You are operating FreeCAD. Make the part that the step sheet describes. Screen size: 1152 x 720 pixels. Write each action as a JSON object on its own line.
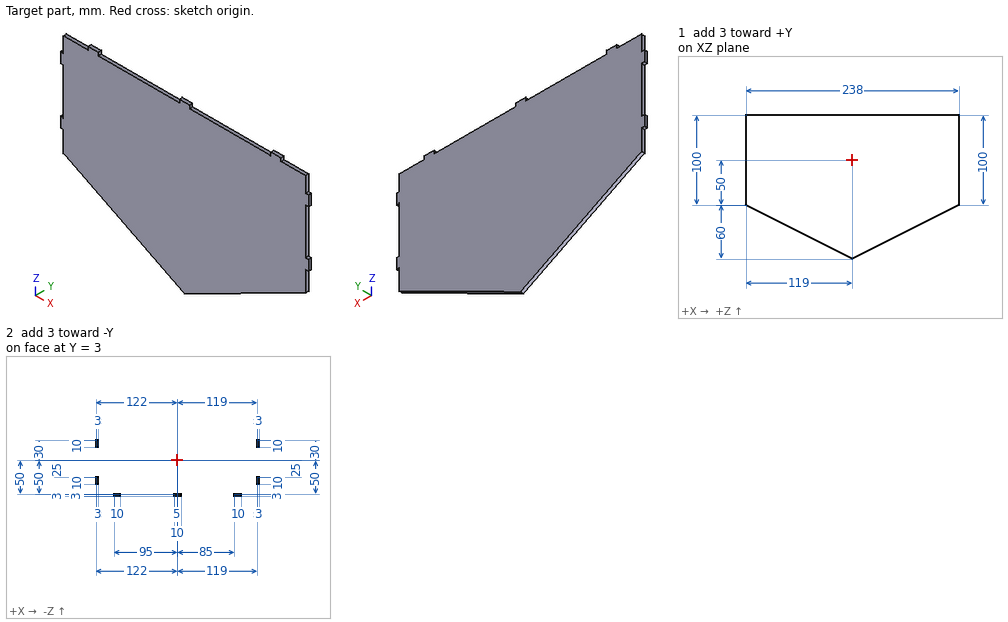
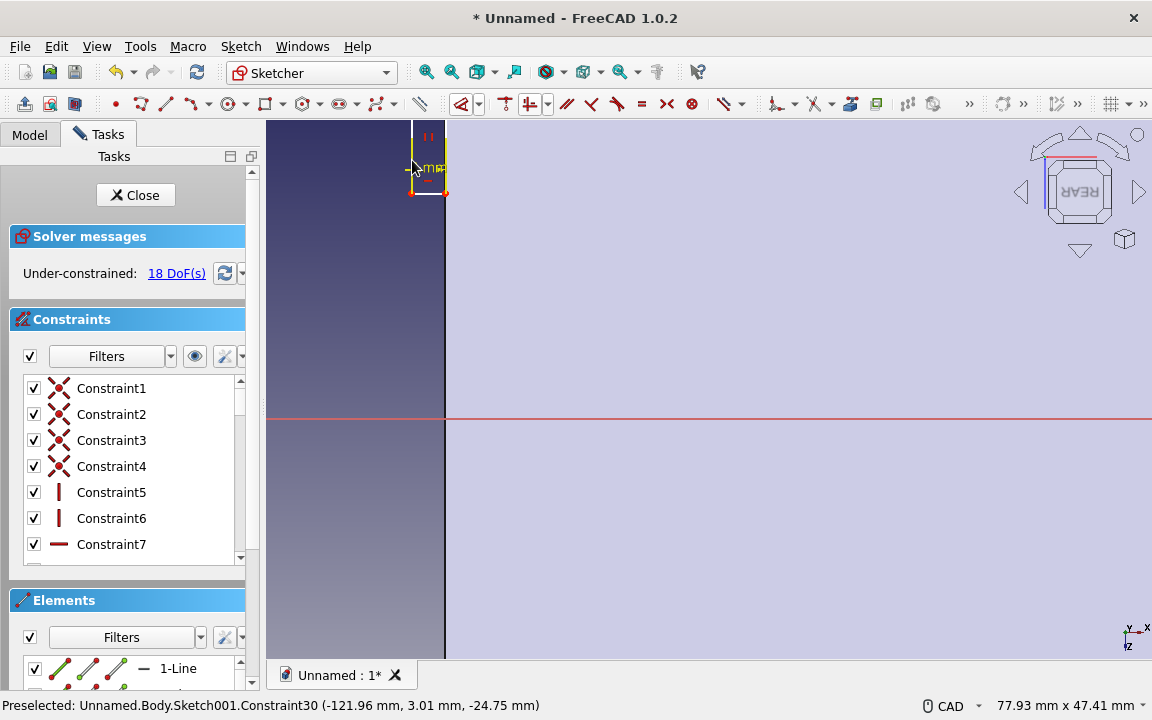
{"action": "left_click", "coordinate": [412, 159]}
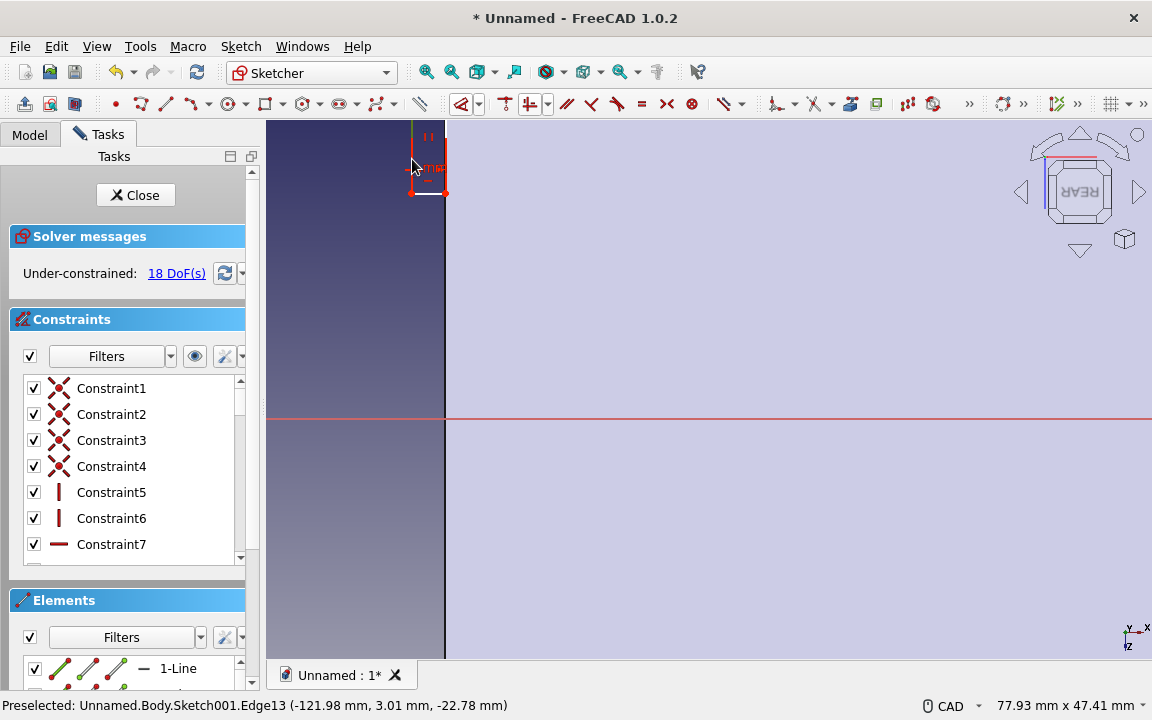
{"action": "key", "text": "i"}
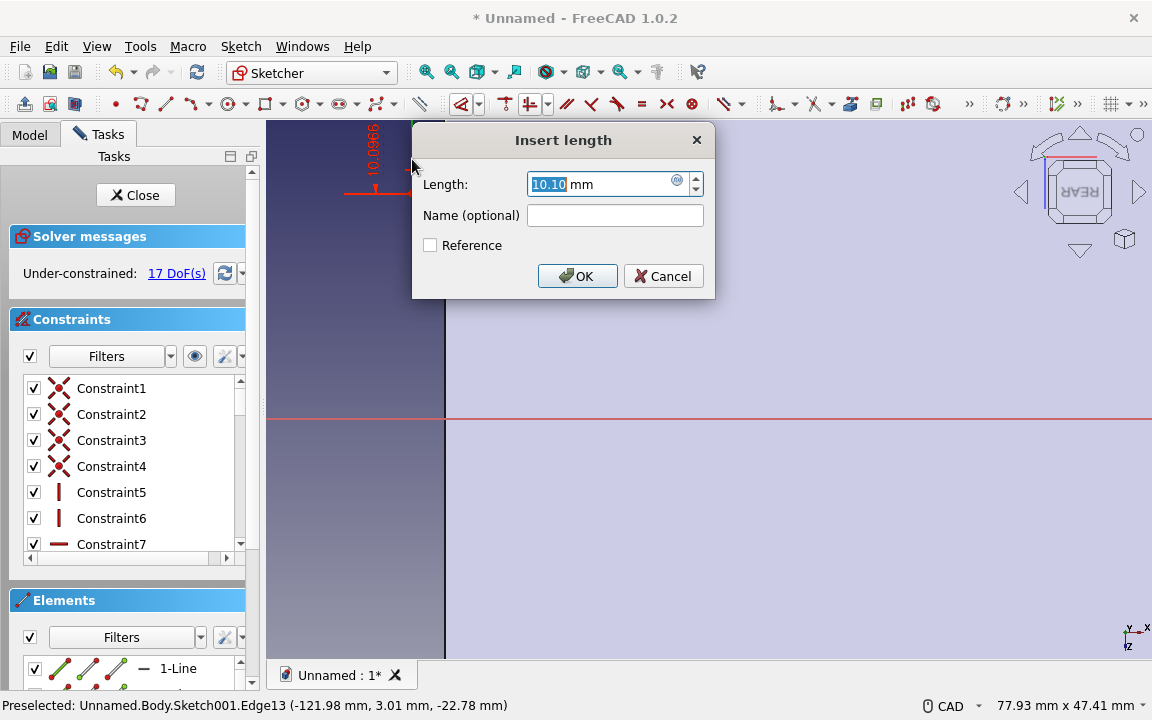
{"action": "type", "text": "10"}
{"action": "key", "text": "Return"}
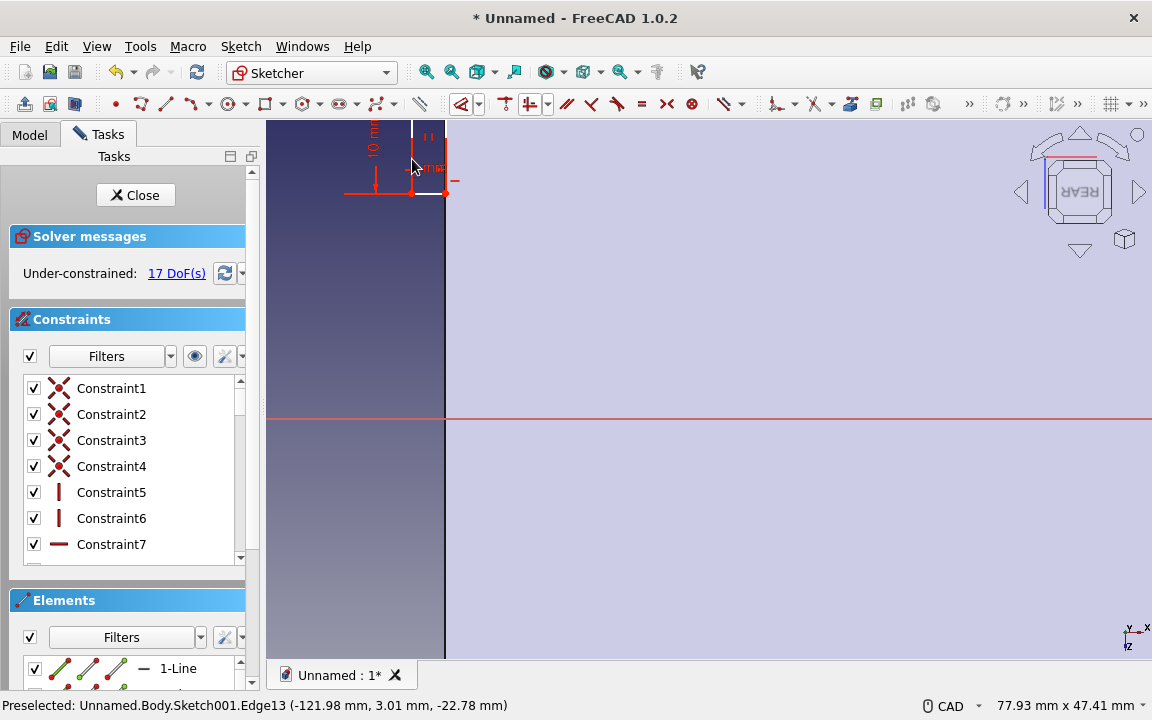
{"action": "scroll", "coordinate": [411, 358], "scroll_direction": "down", "scroll_amount": 9}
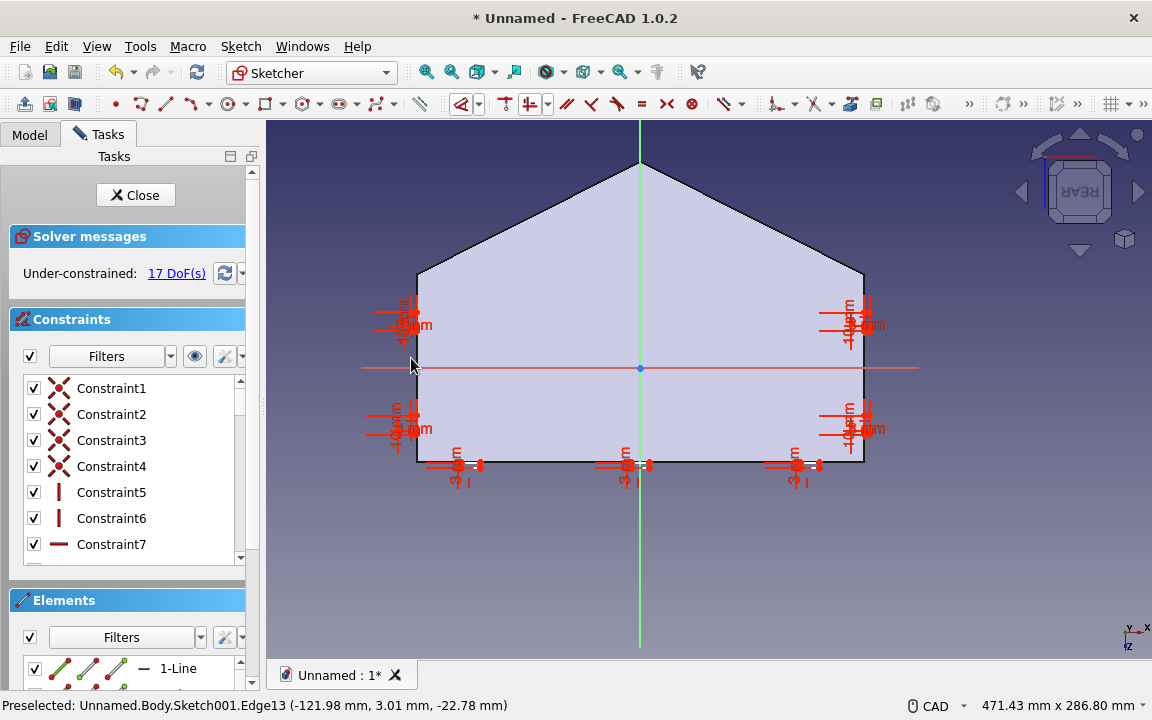
{"action": "scroll", "coordinate": [468, 468], "scroll_direction": "up", "scroll_amount": 5}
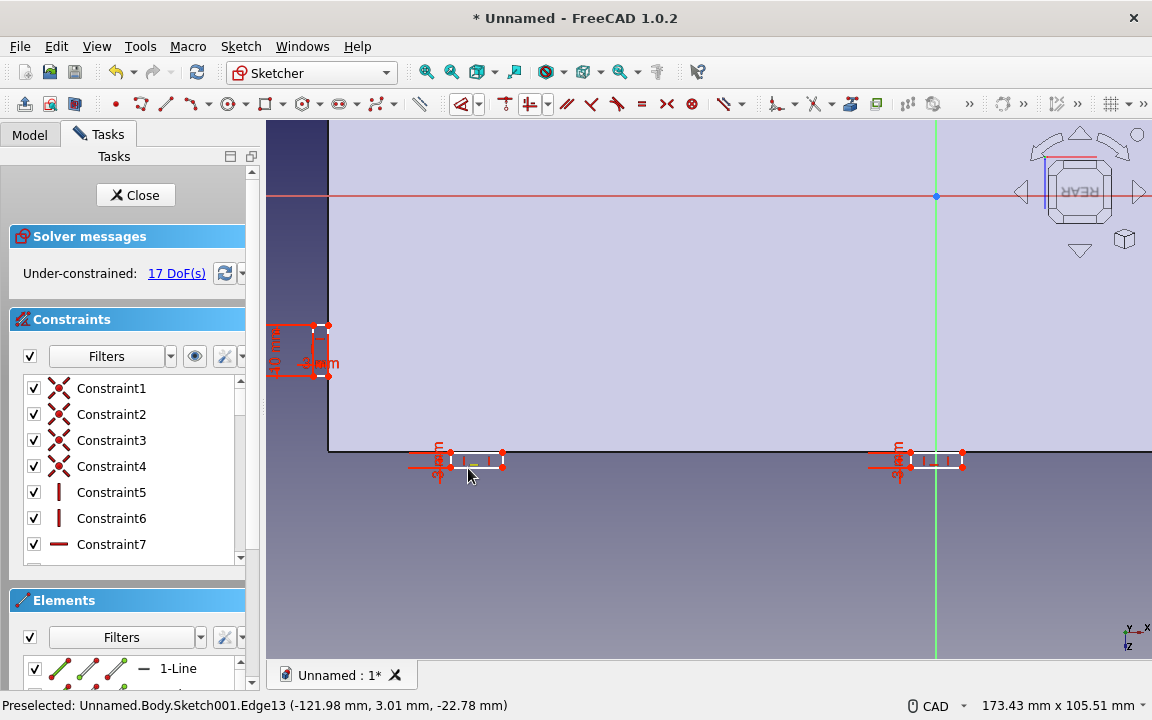
{"action": "left_click", "coordinate": [466, 468]}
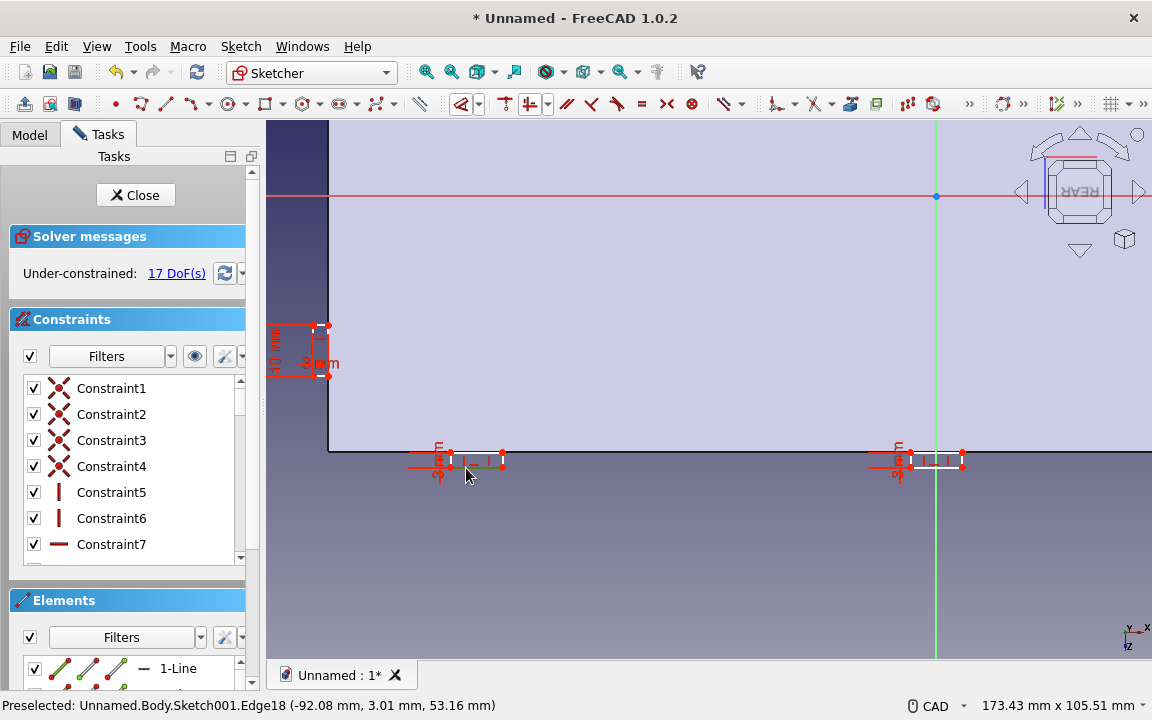
{"action": "key", "text": "l"}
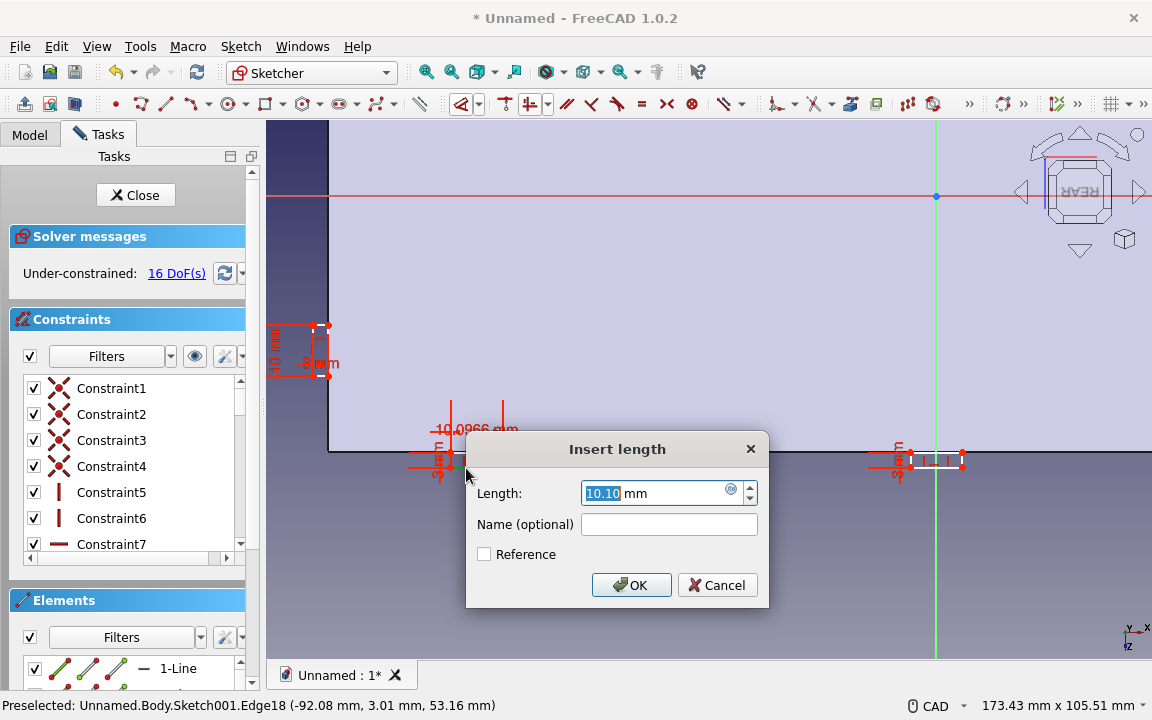
{"action": "type", "text": "10"}
{"action": "key", "text": "Return"}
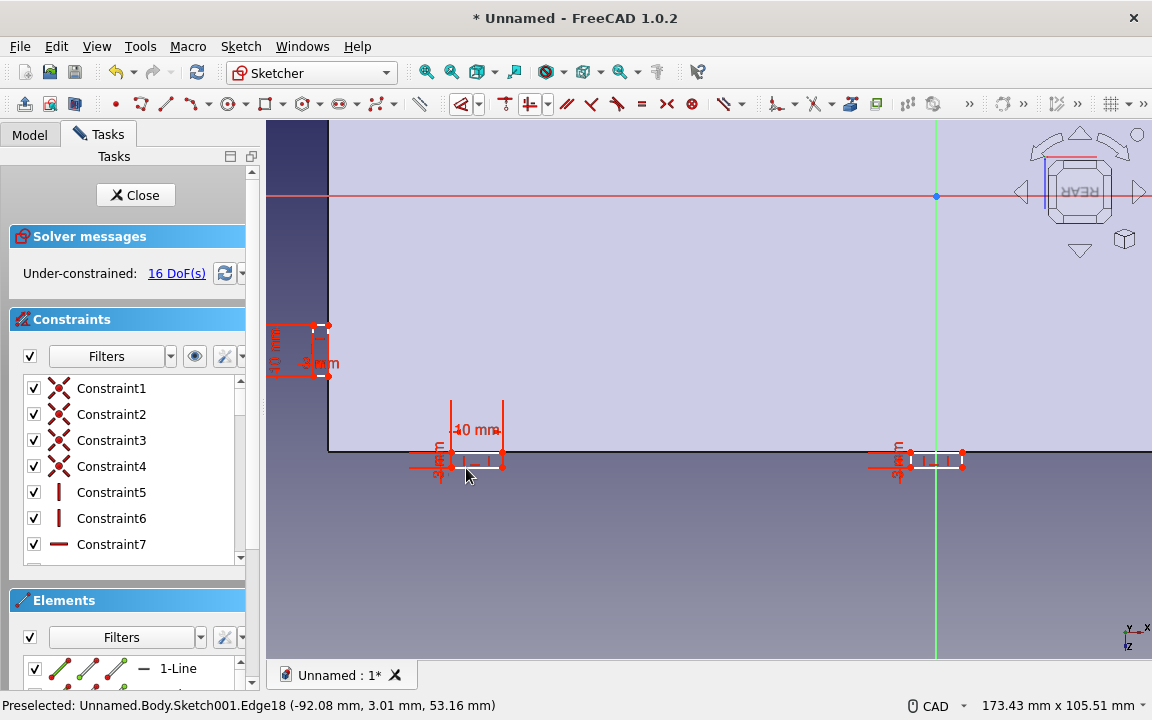
{"action": "scroll", "coordinate": [468, 468], "scroll_direction": "down", "scroll_amount": 5}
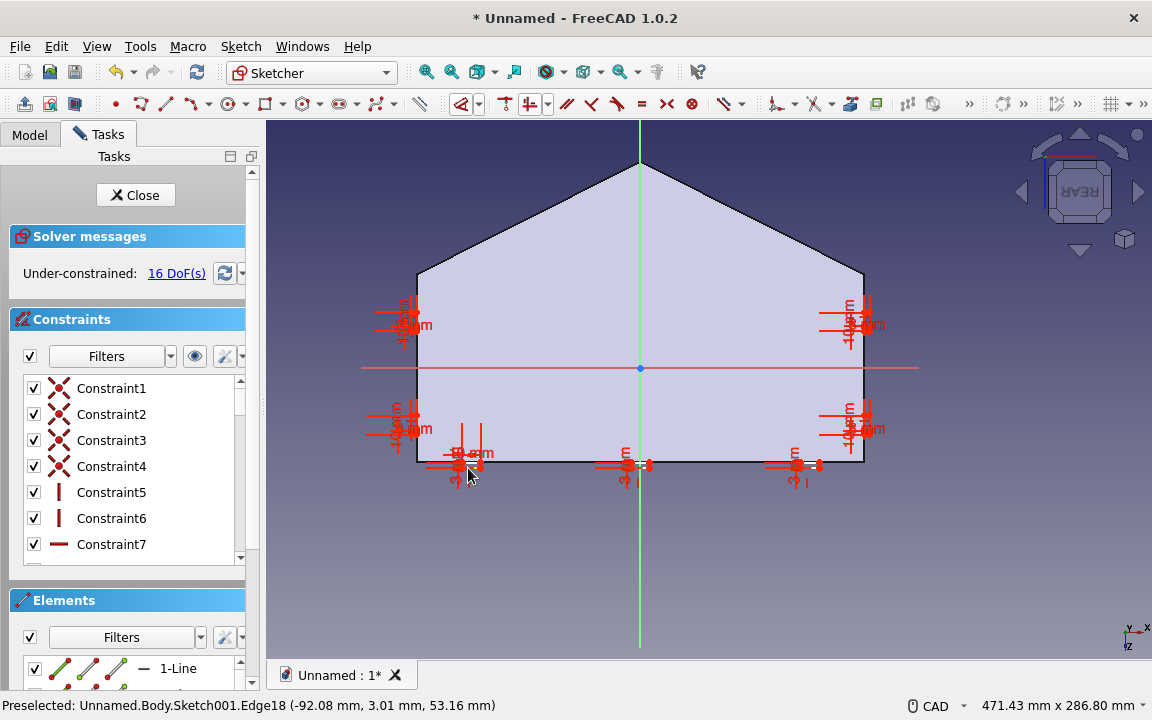
{"action": "scroll", "coordinate": [806, 468], "scroll_direction": "up", "scroll_amount": 5}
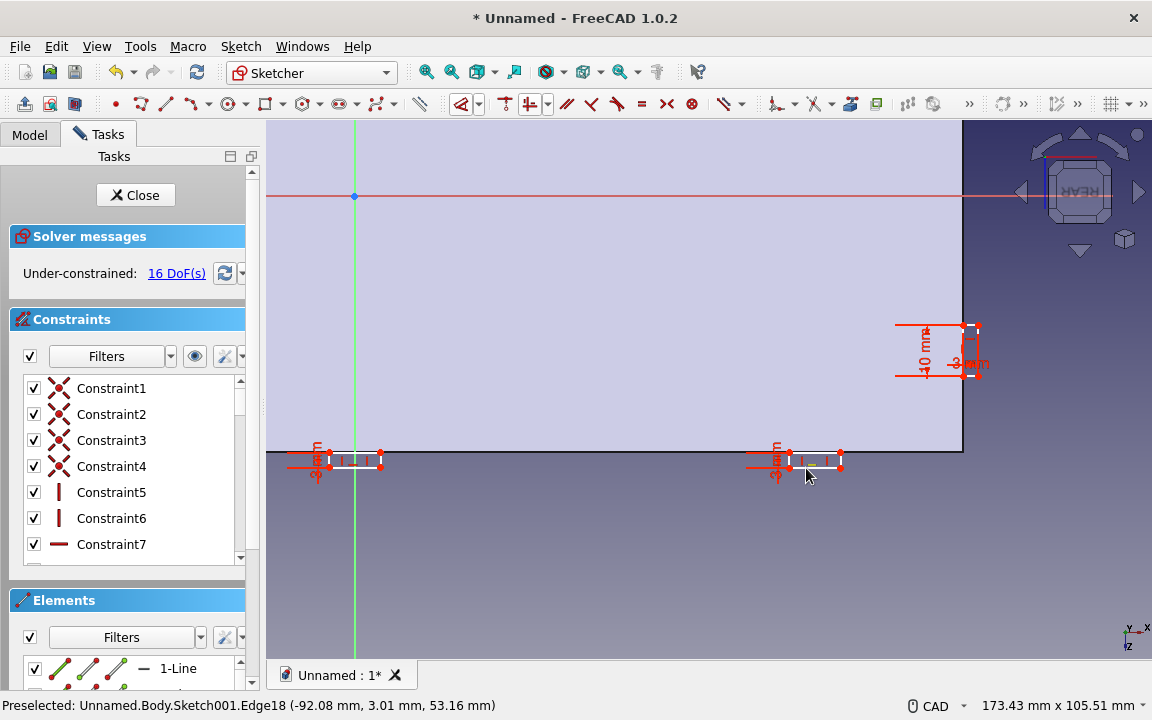
{"action": "left_click", "coordinate": [805, 468]}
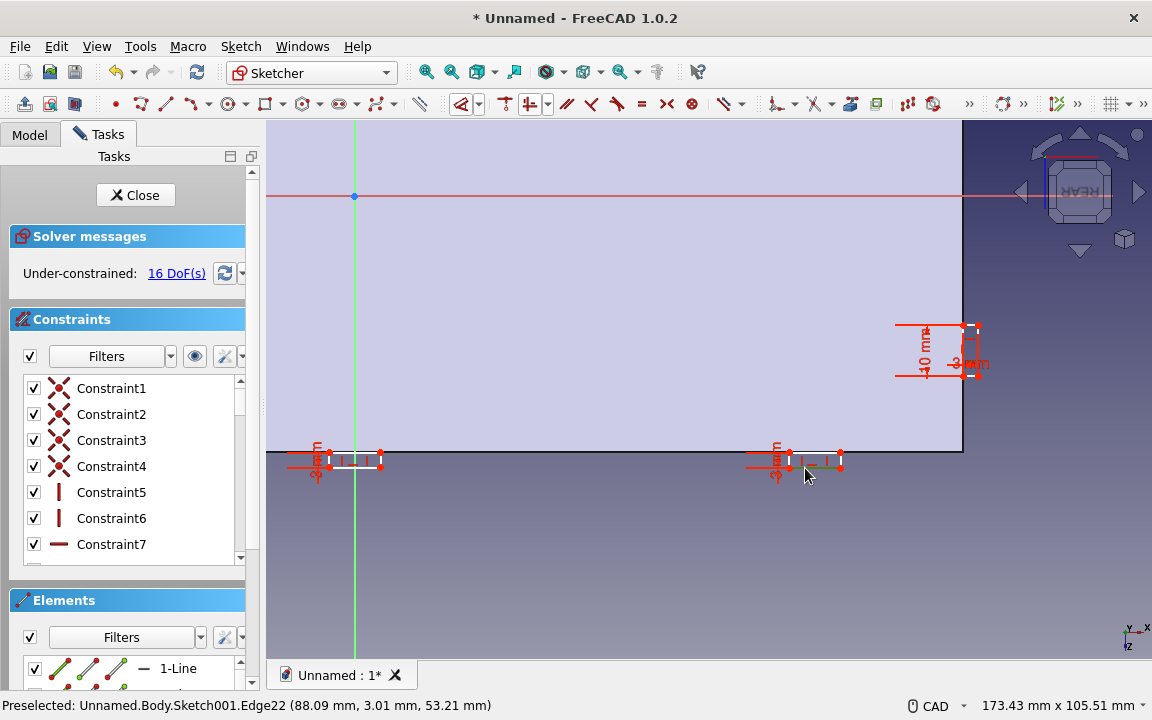
{"action": "key", "text": "l"}